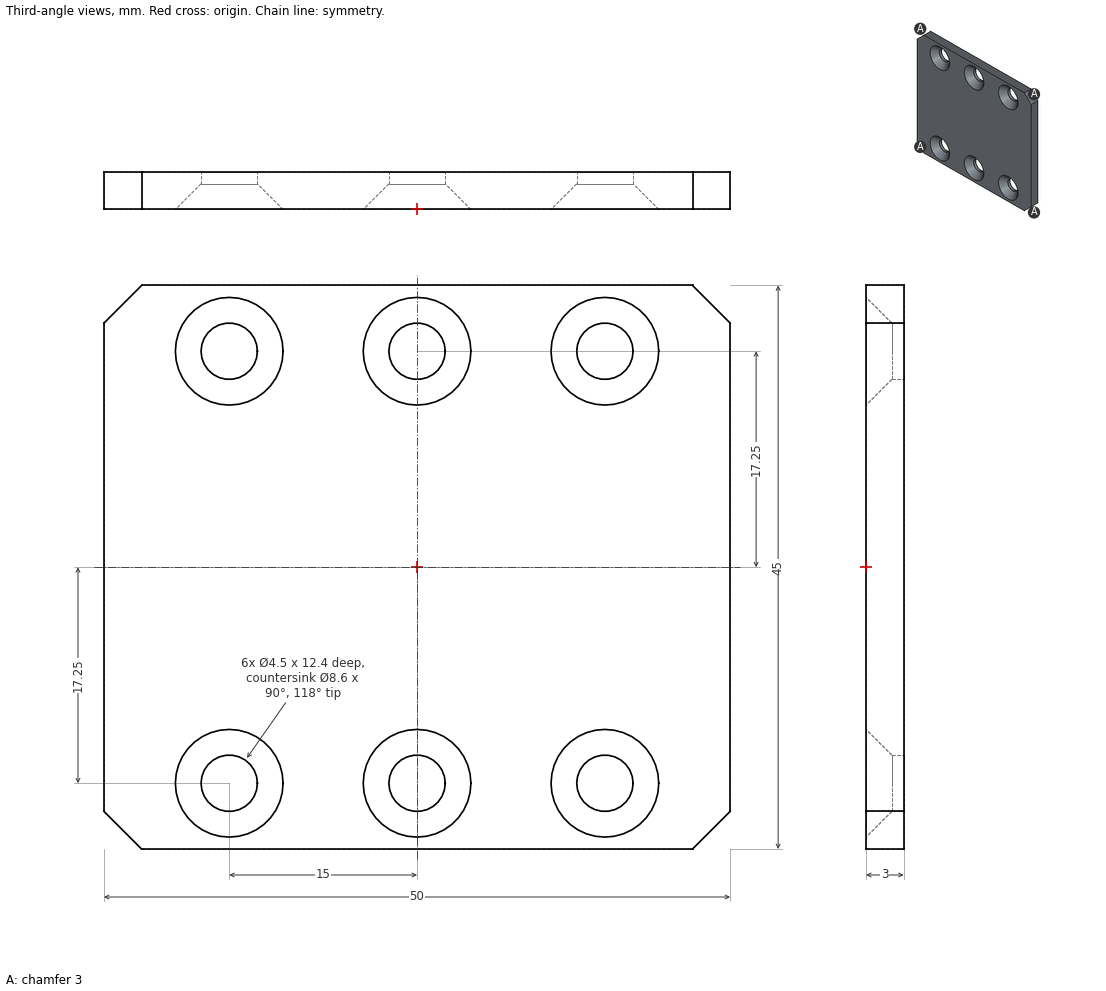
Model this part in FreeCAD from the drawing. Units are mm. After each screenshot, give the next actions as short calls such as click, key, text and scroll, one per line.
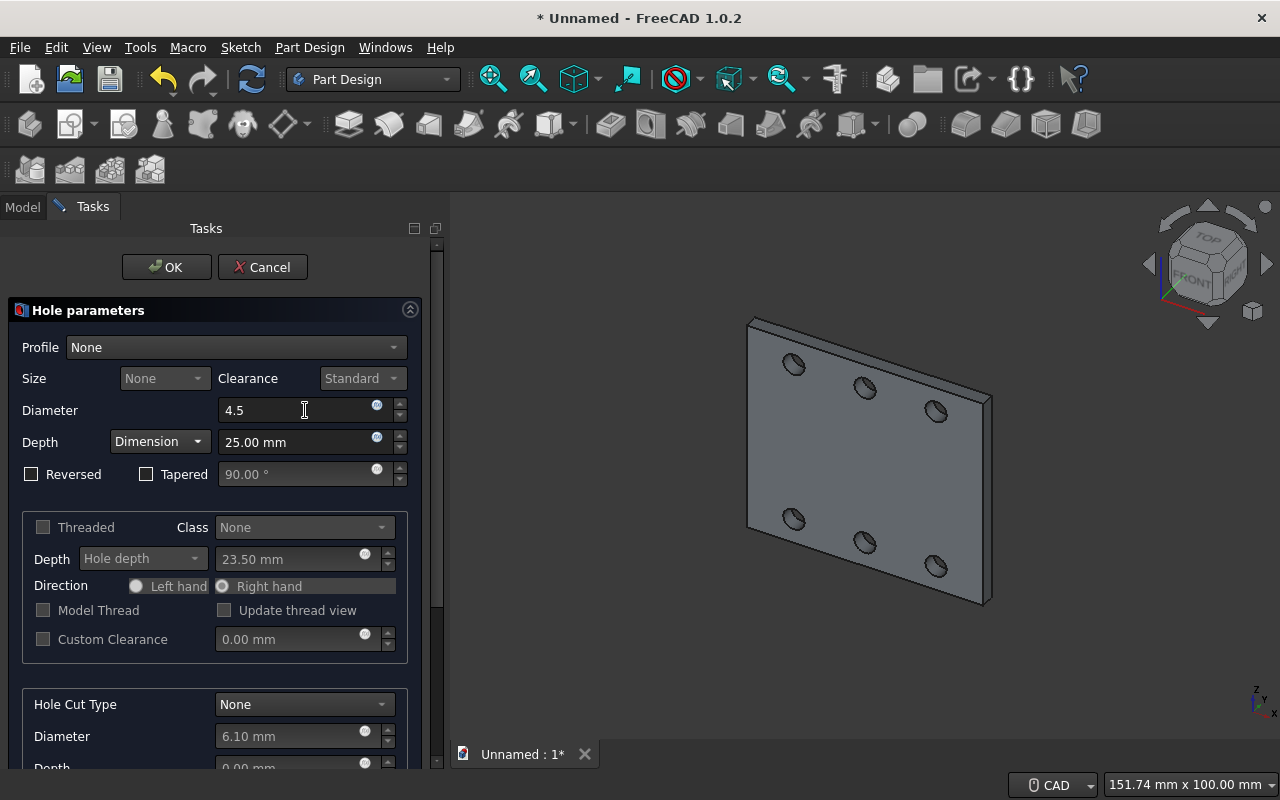
triple_click(305, 442)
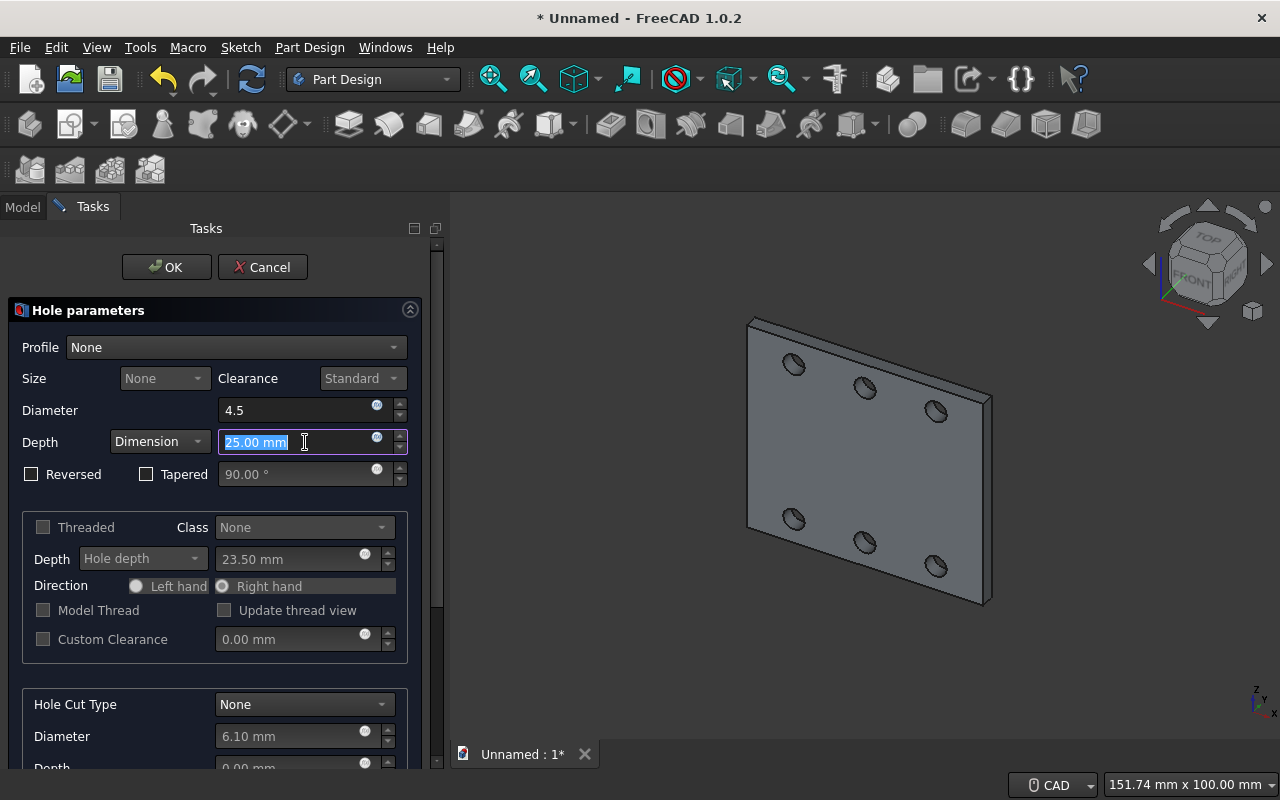
text(12.4)
key(Tab)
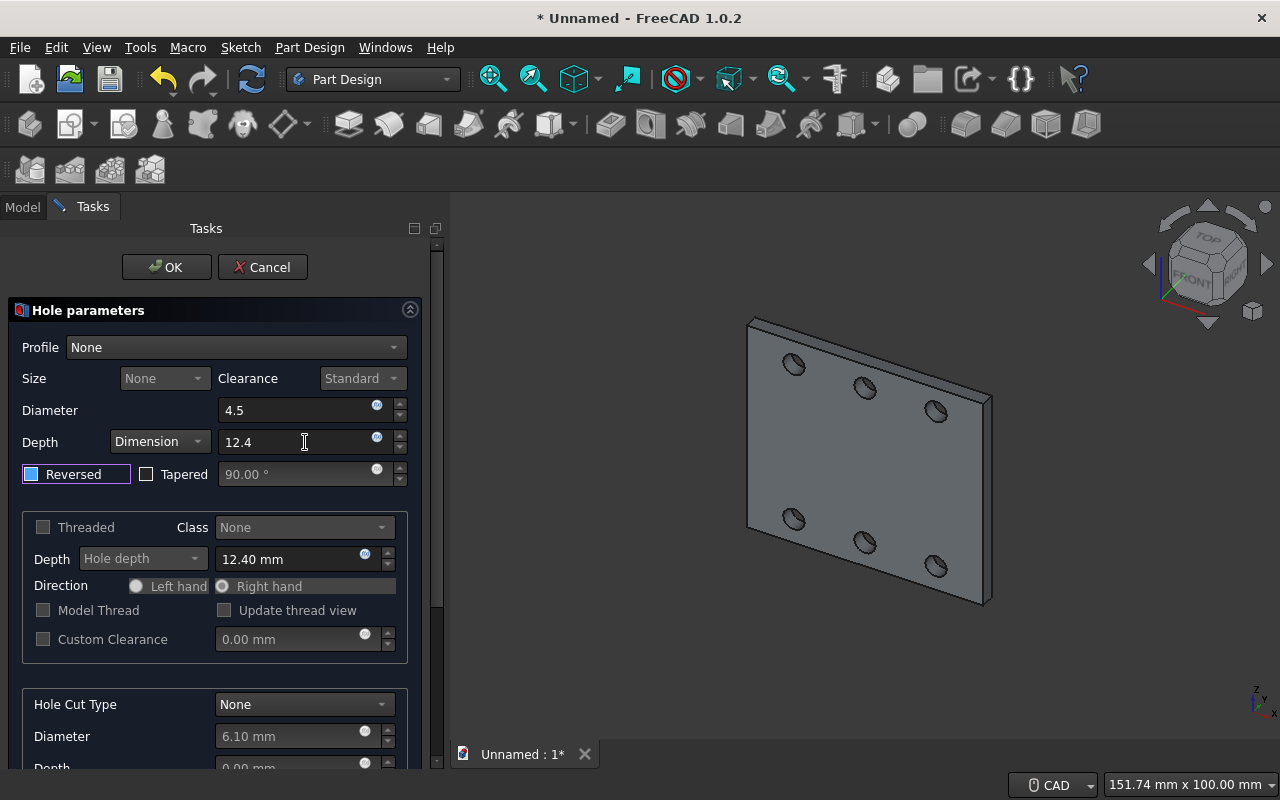
click(306, 704)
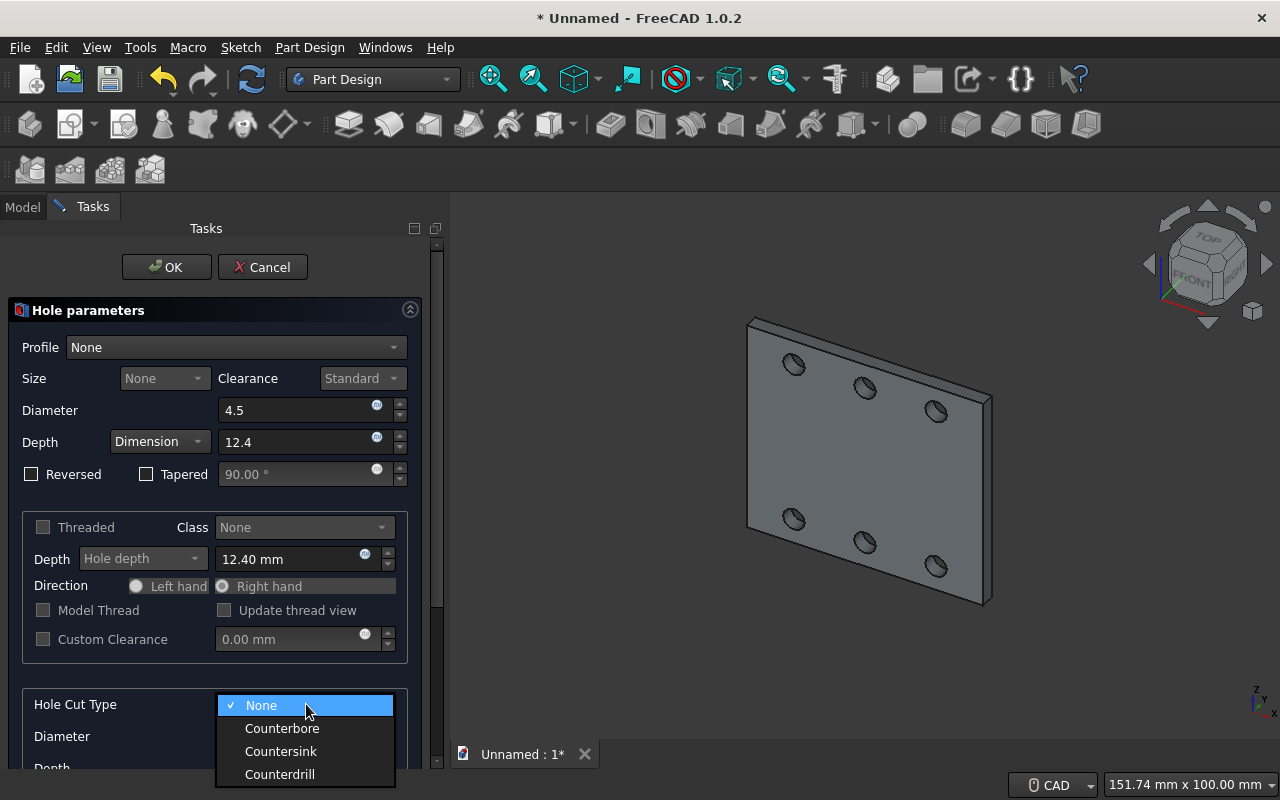
click(304, 752)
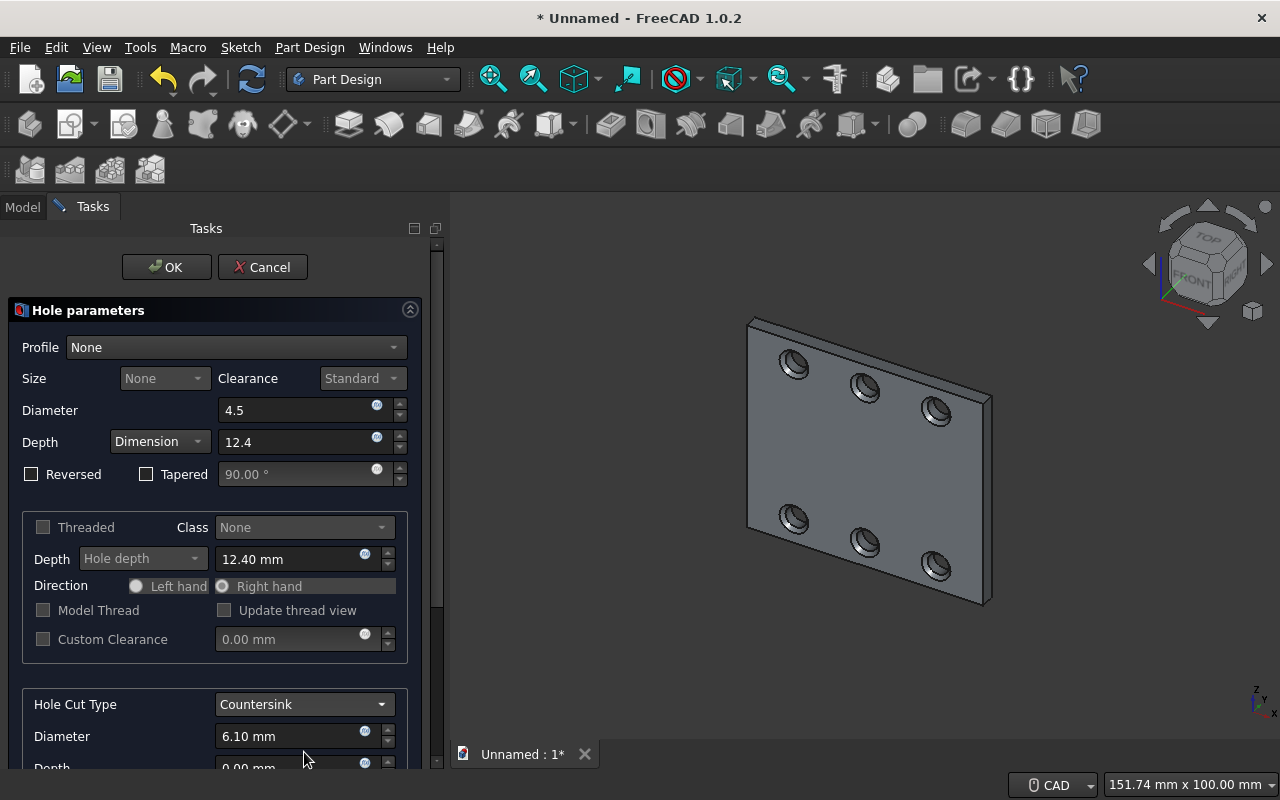
triple_click(298, 736)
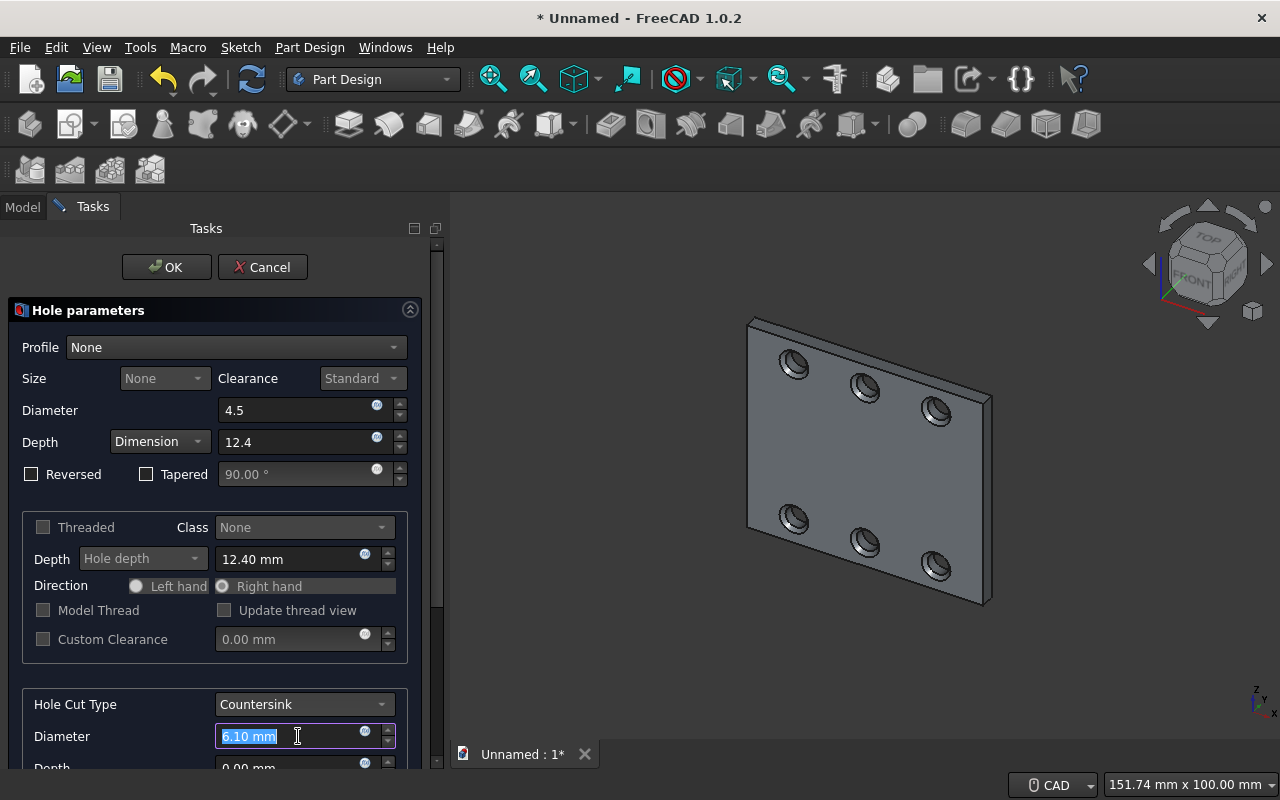
text(8.6)
key(Tab)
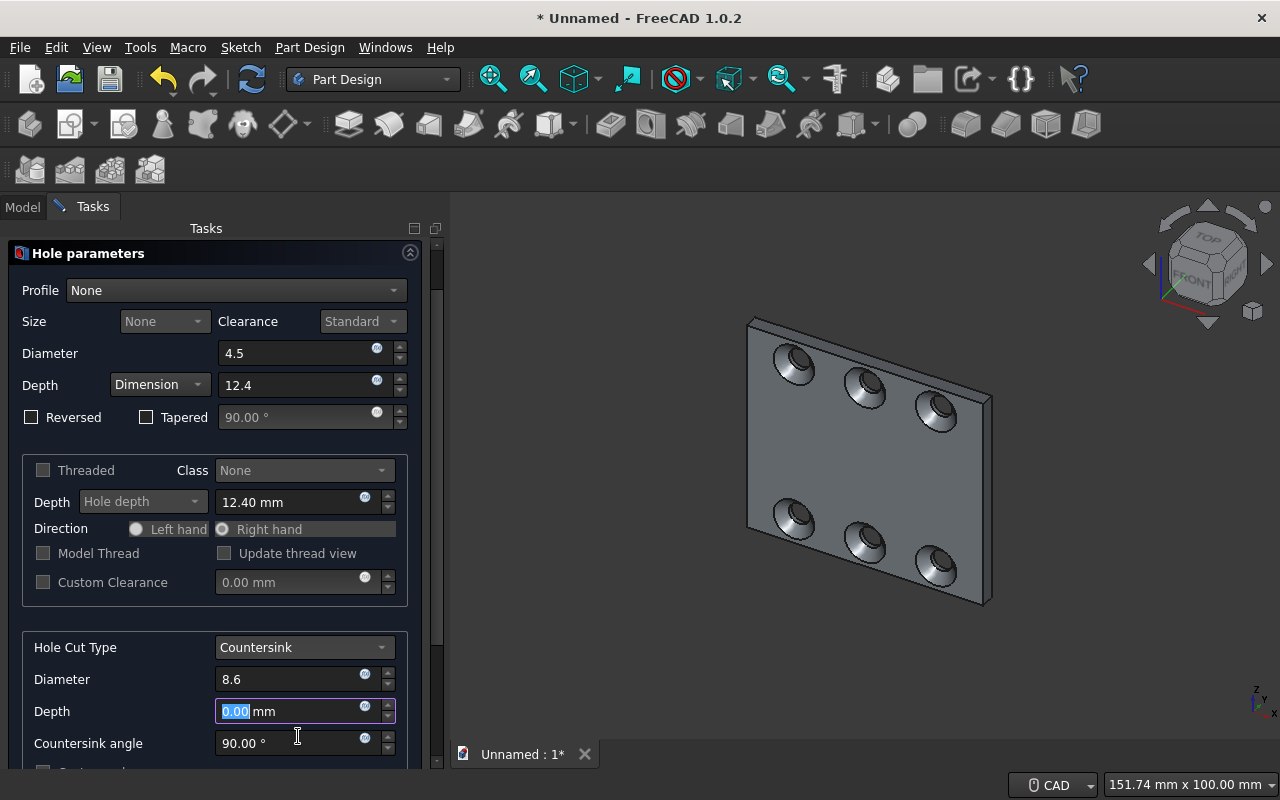
scroll(437, 503, up, 2)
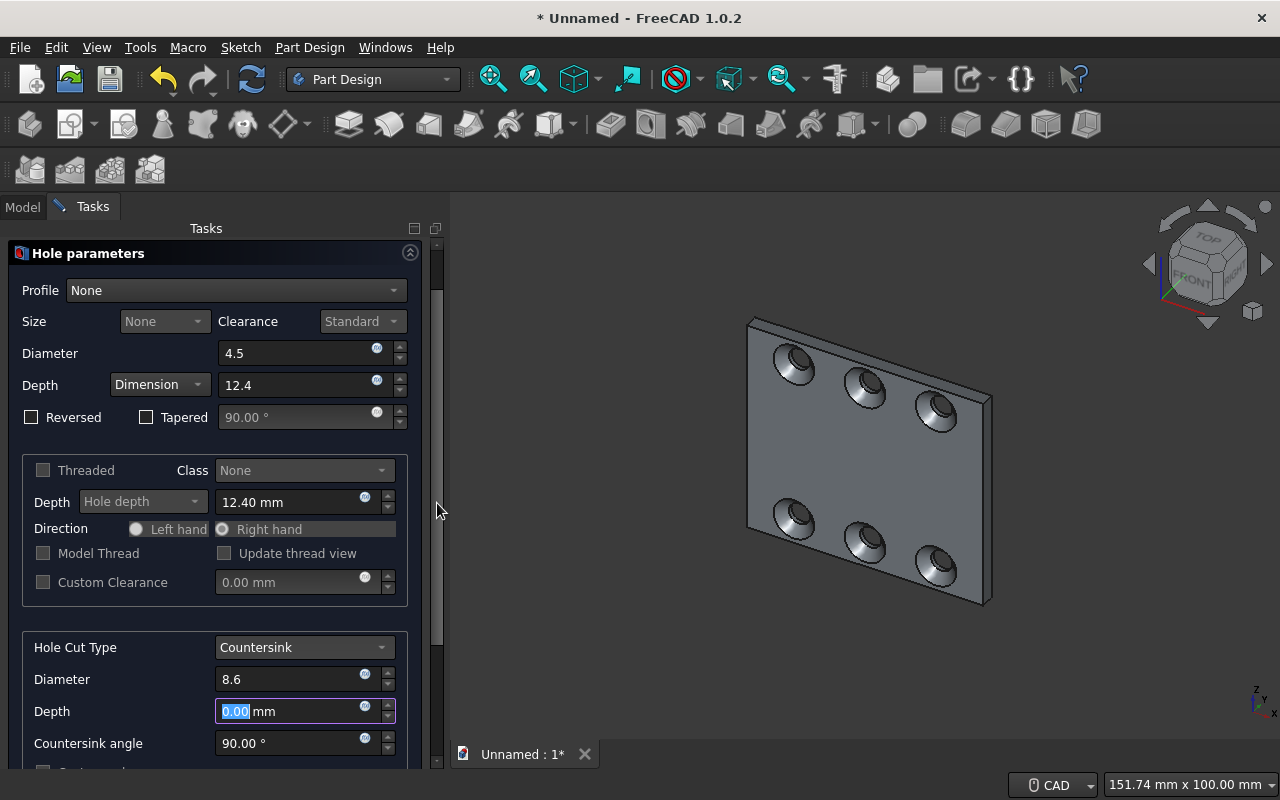
click(167, 267)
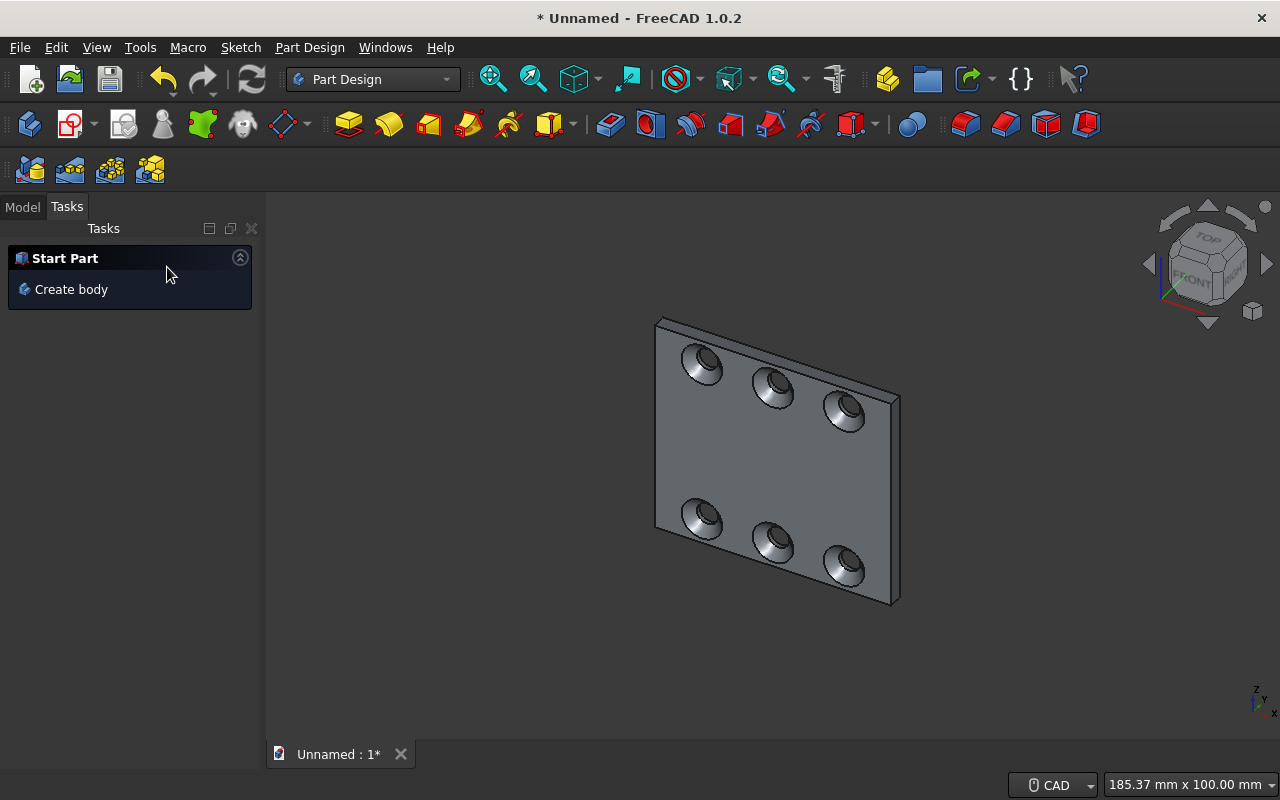
click(896, 398)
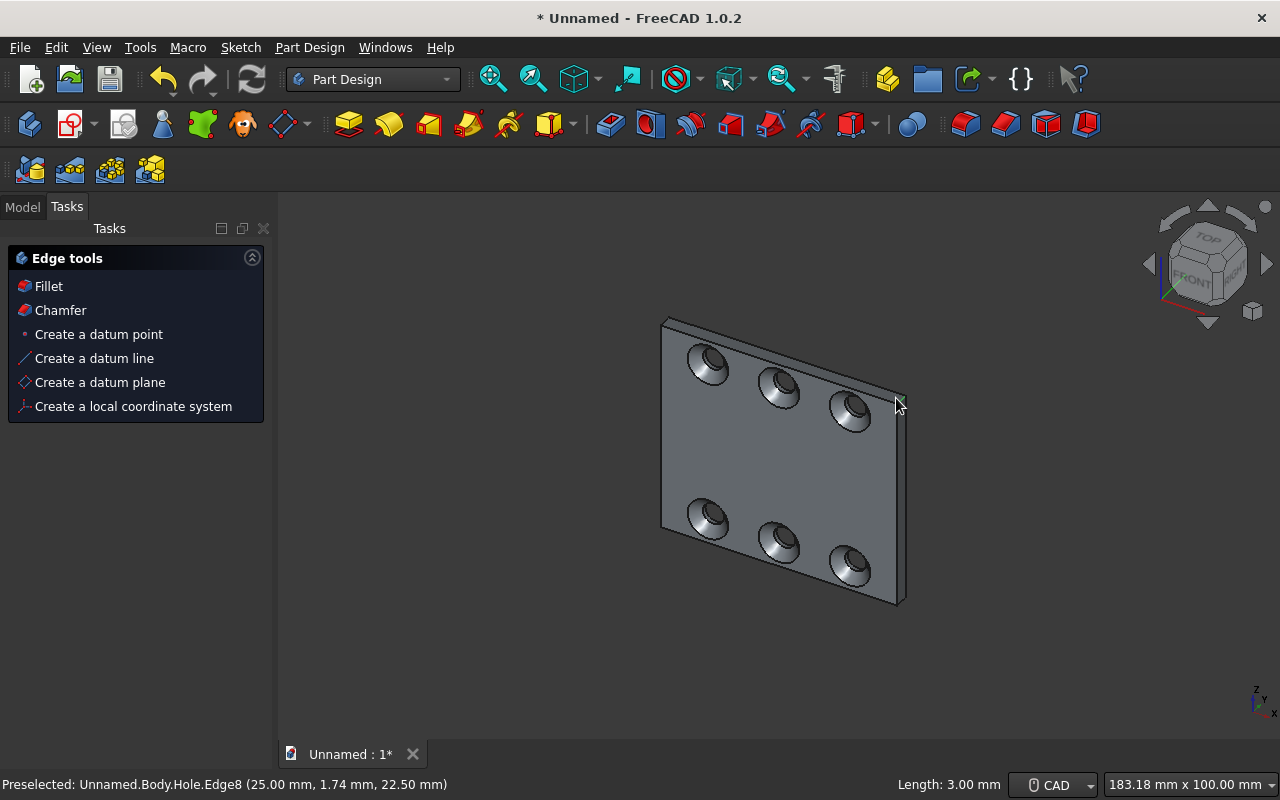
scroll(665, 320, up, 5)